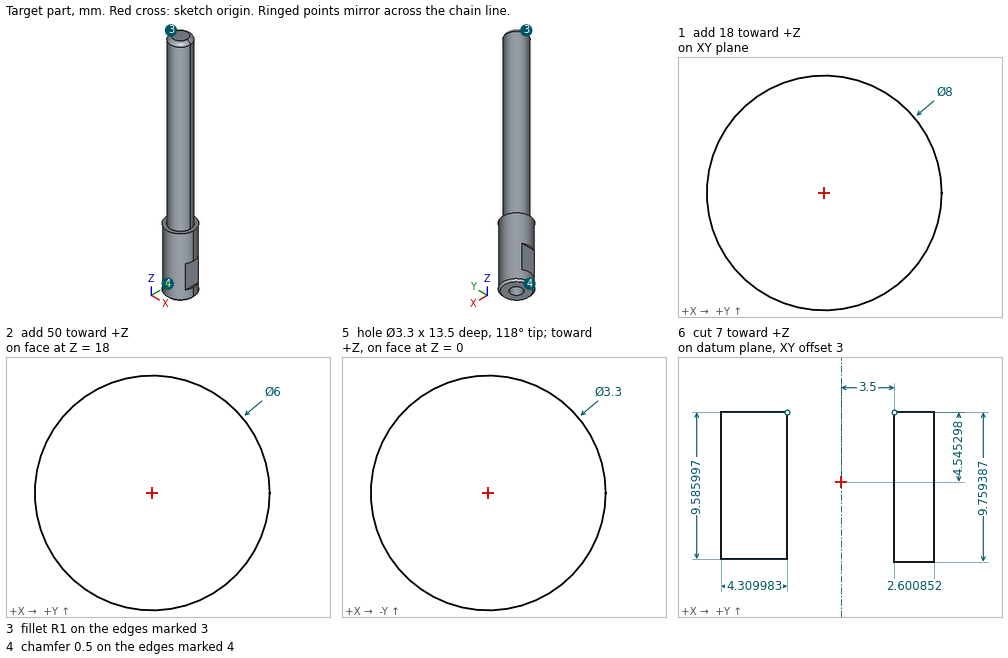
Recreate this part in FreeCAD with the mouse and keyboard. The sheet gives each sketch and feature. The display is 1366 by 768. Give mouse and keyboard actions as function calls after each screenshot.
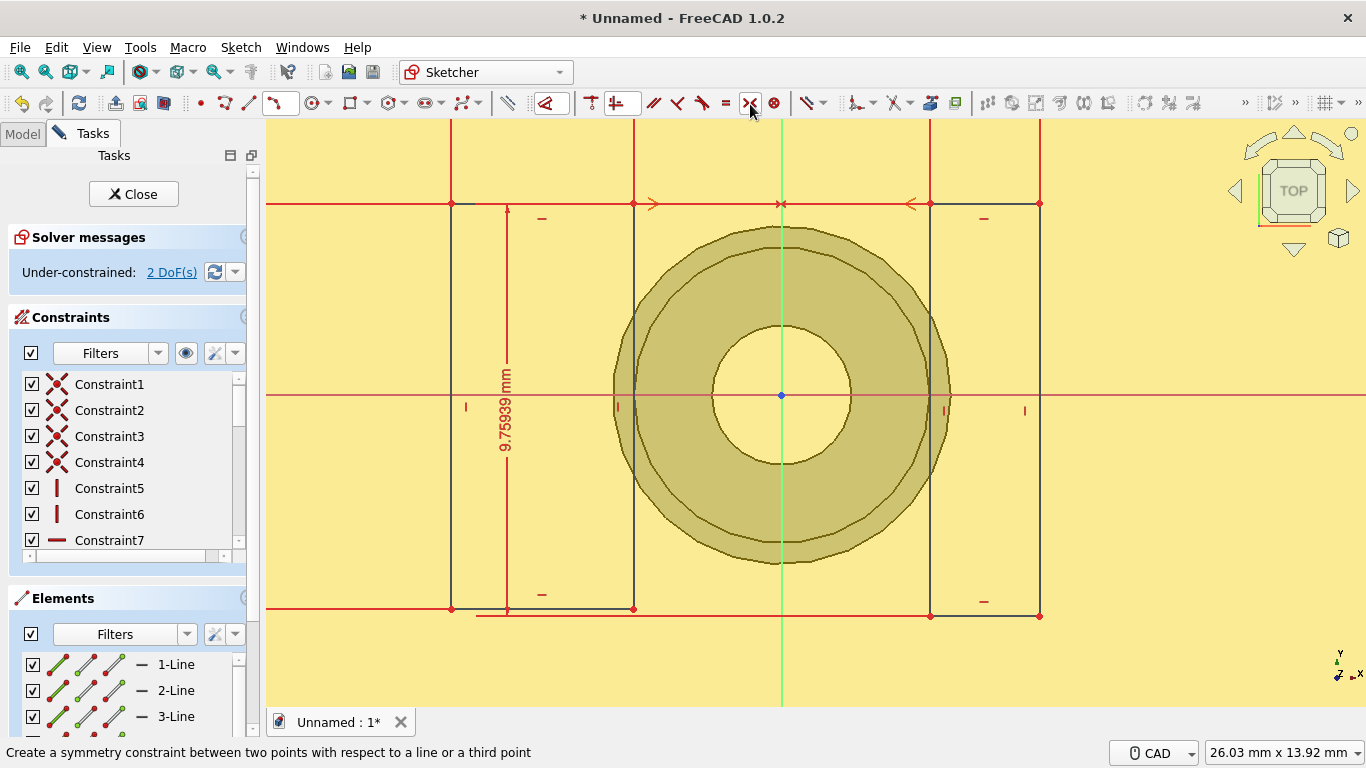
click(546, 104)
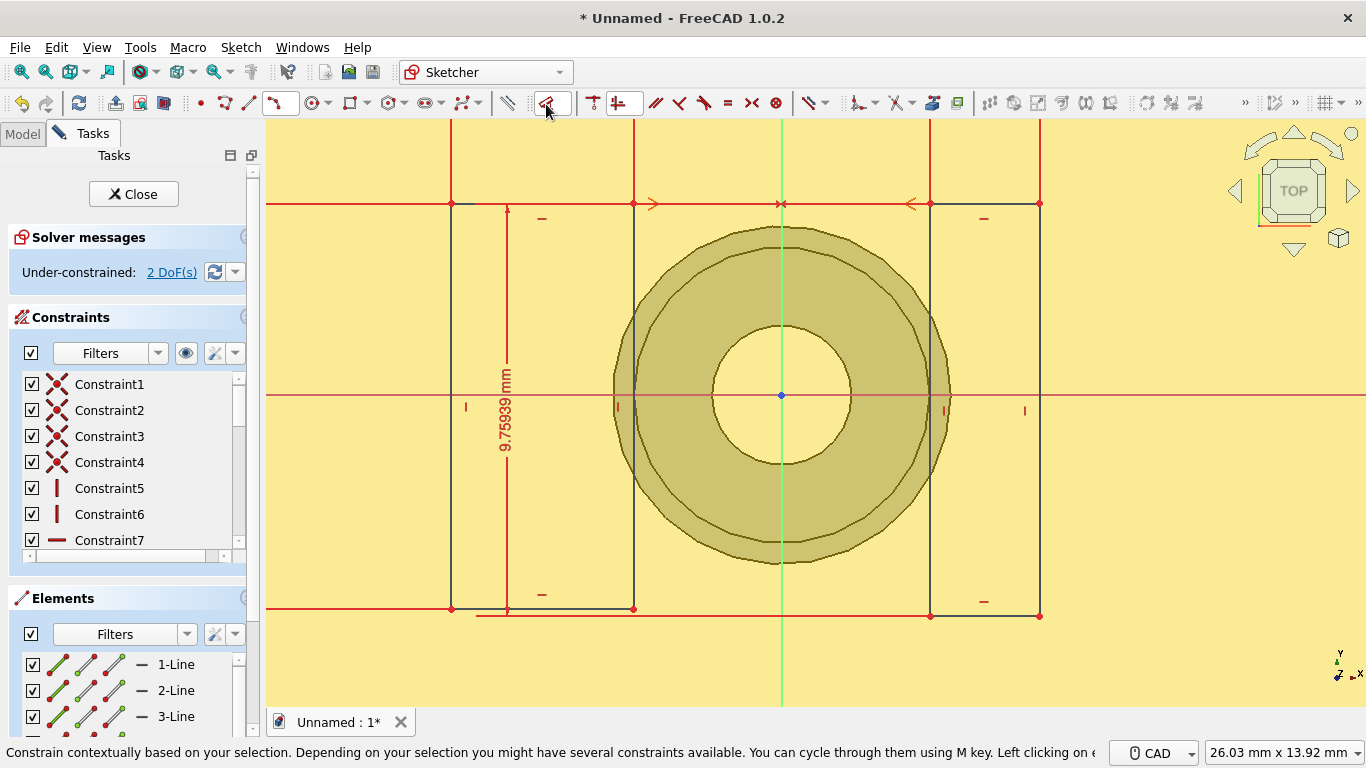
click(930, 204)
click(856, 170)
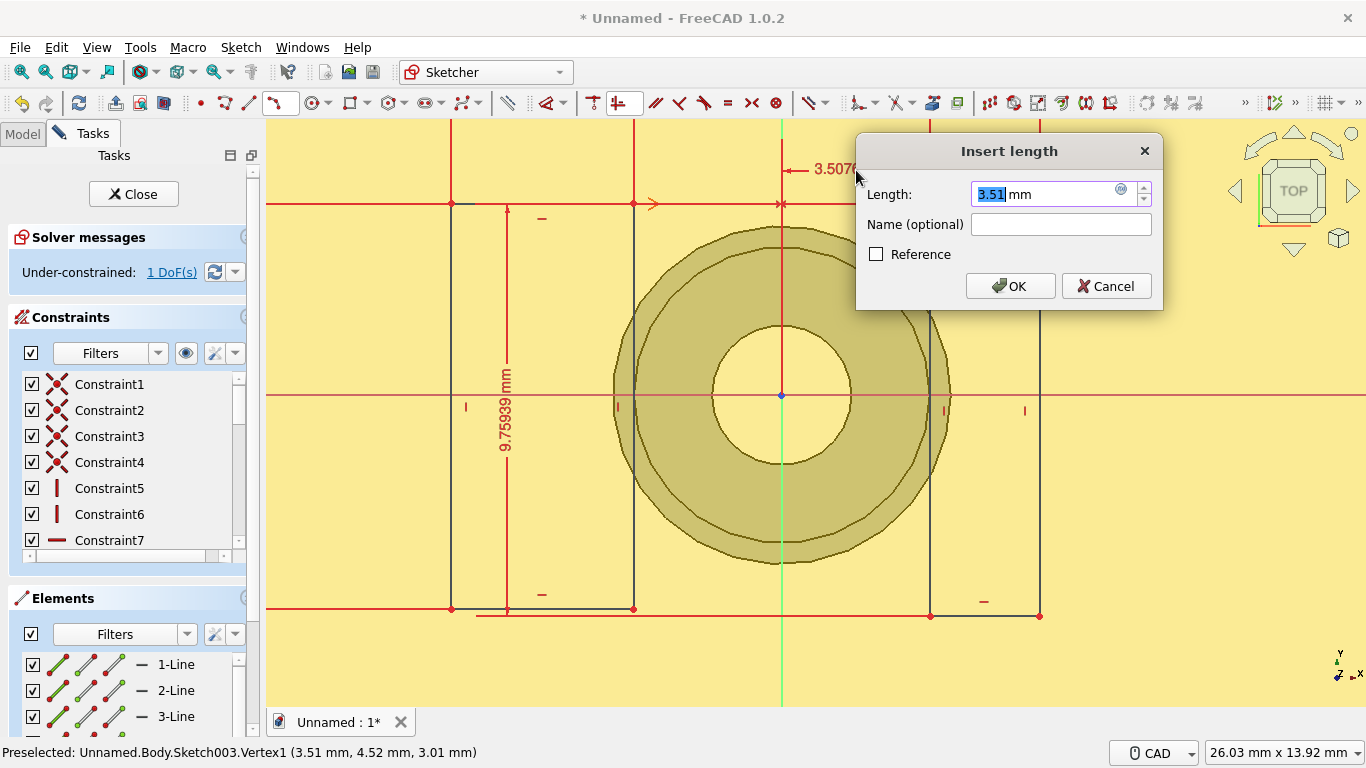
text(3.5)
key(Return)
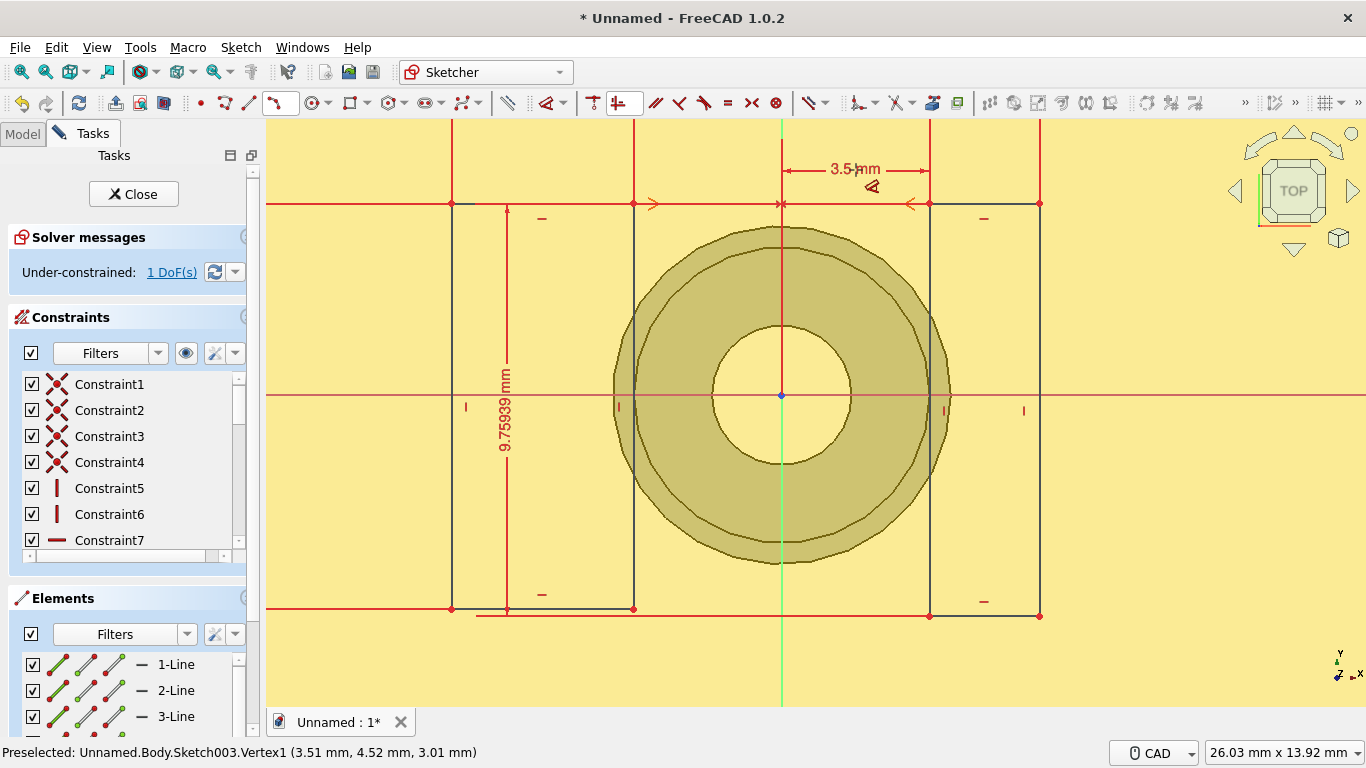
click(930, 204)
click(964, 300)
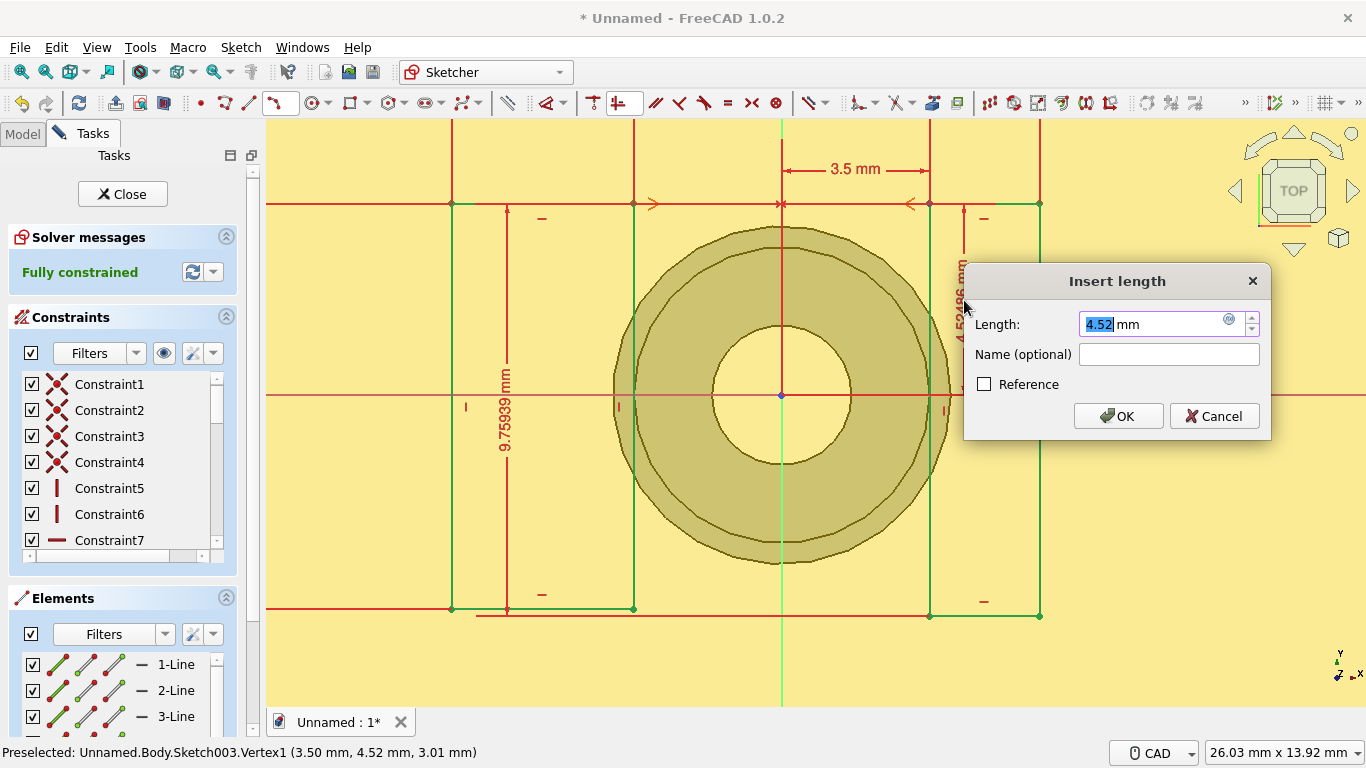
text(4.545298)
key(Return)
key(Escape)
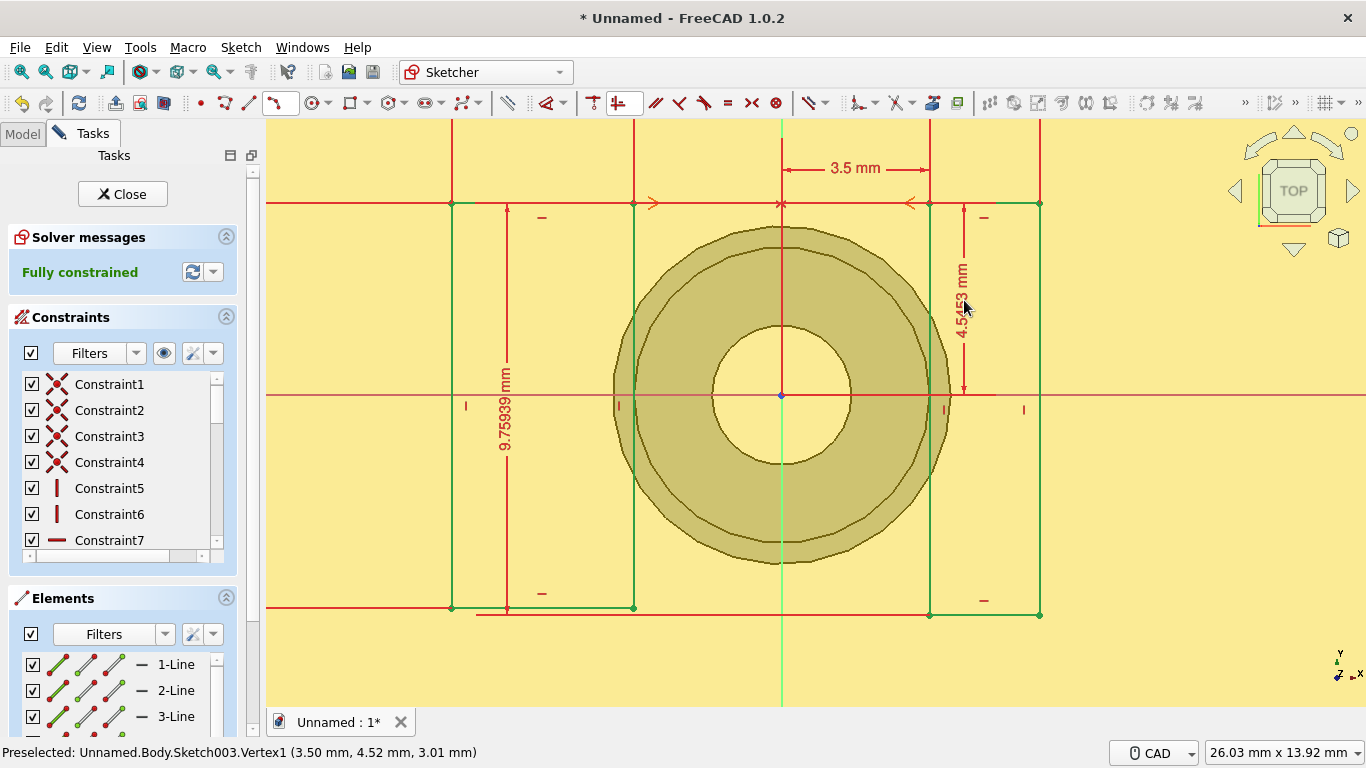
click(123, 194)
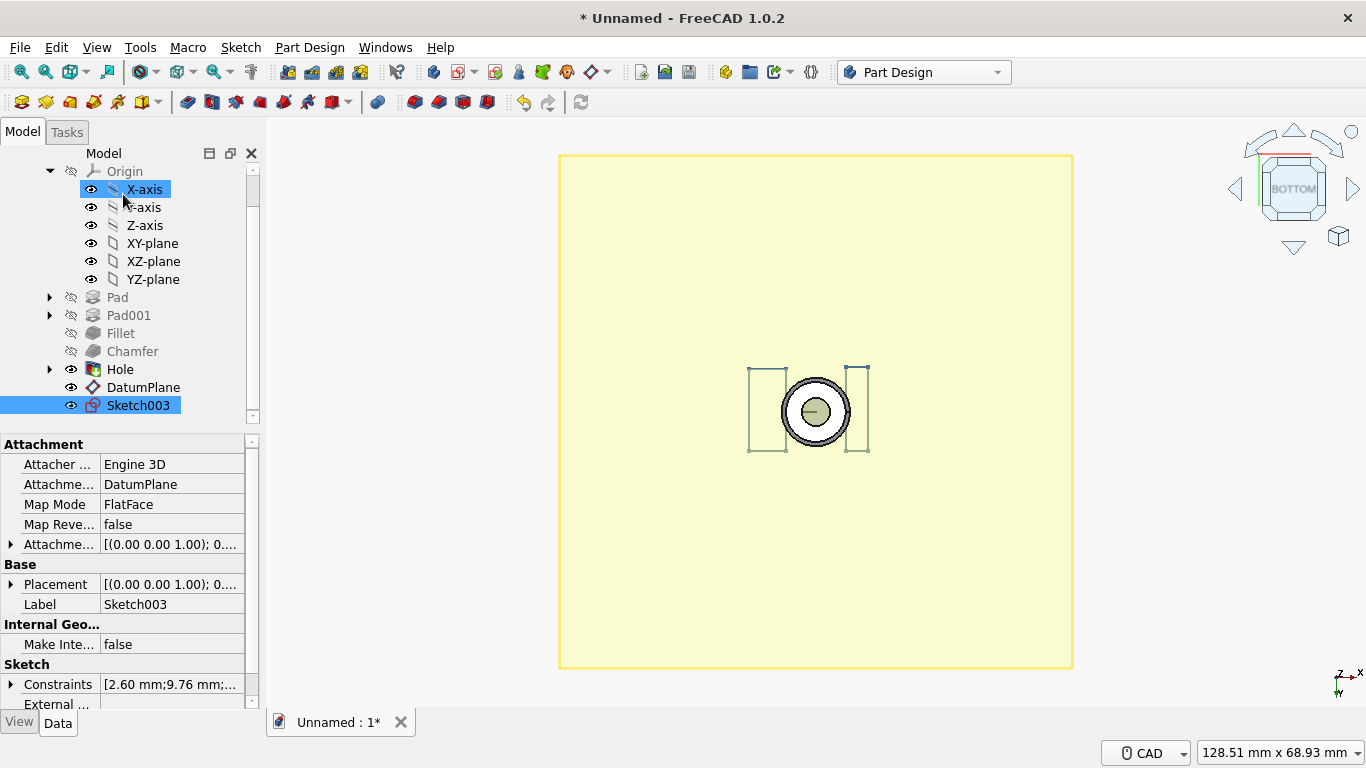
click(188, 102)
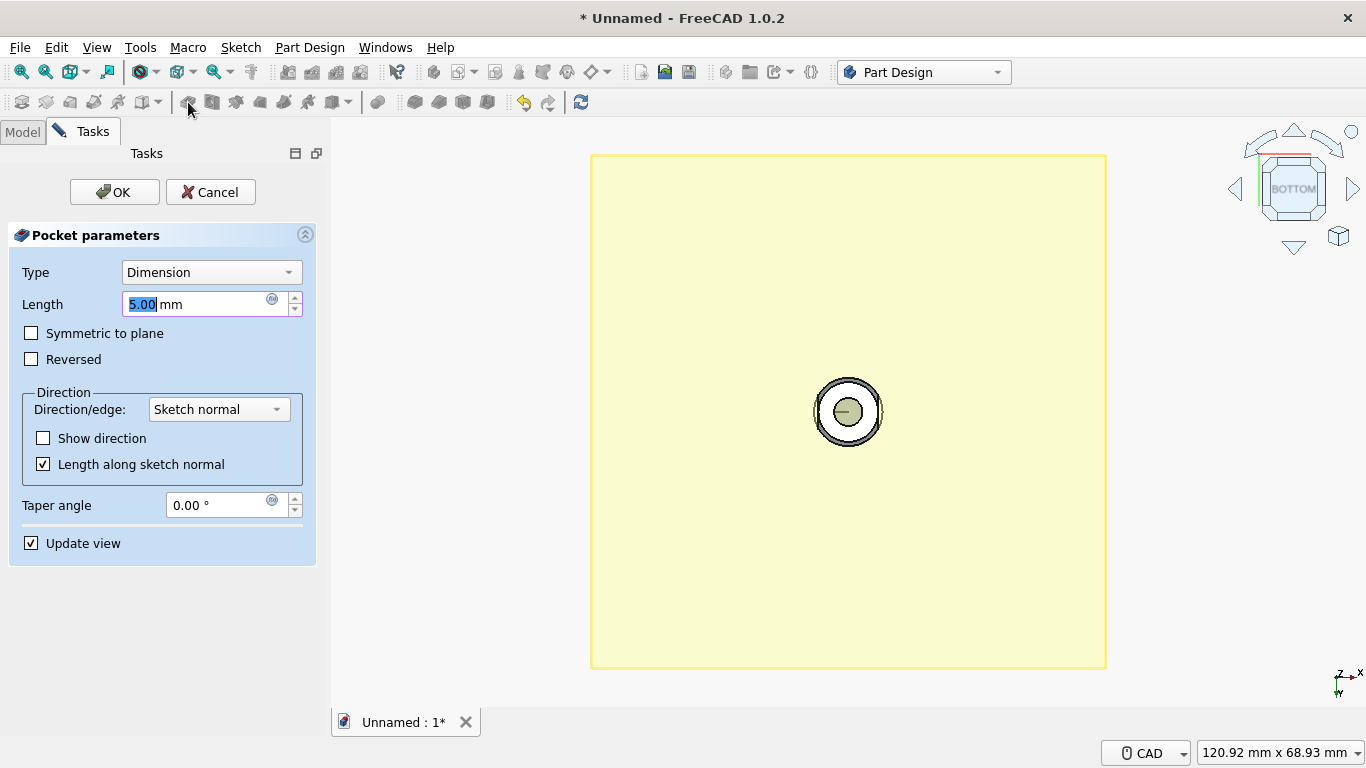
text(7)
key(Tab)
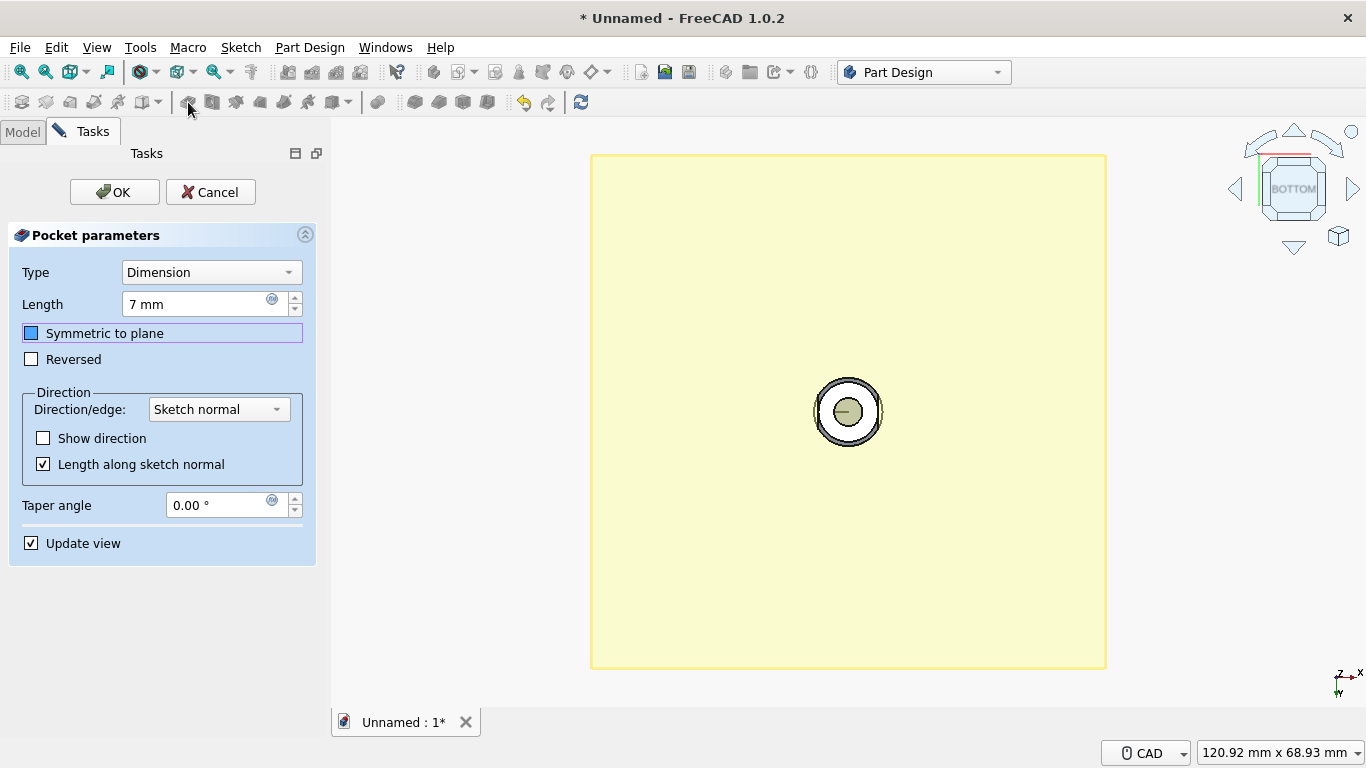
click(30, 359)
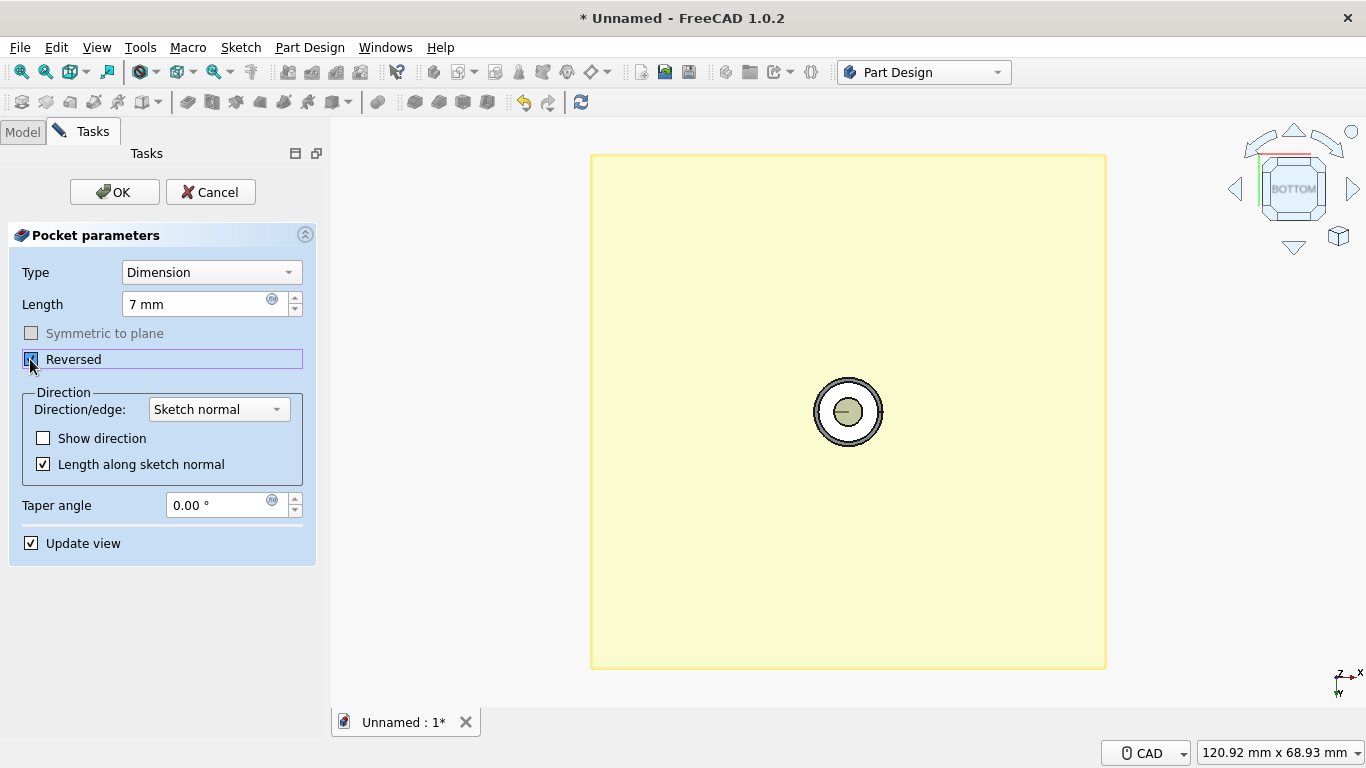
click(115, 192)